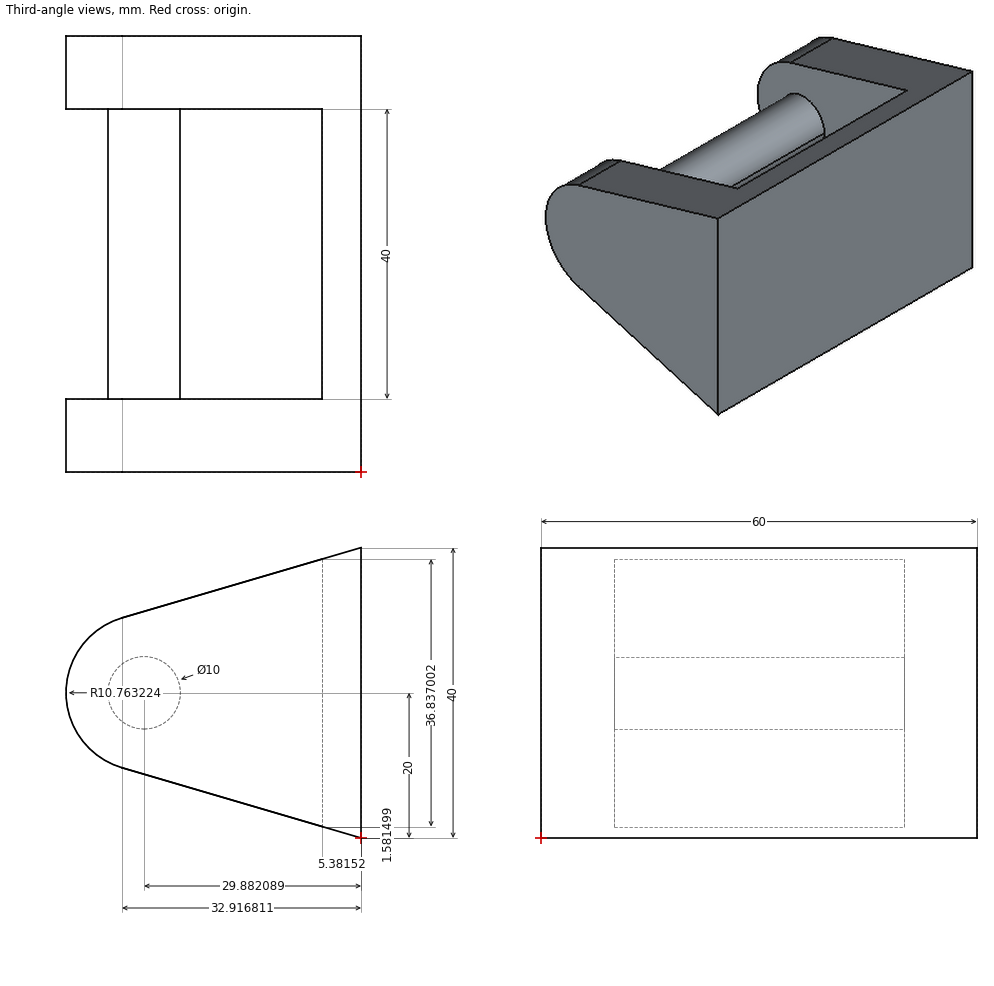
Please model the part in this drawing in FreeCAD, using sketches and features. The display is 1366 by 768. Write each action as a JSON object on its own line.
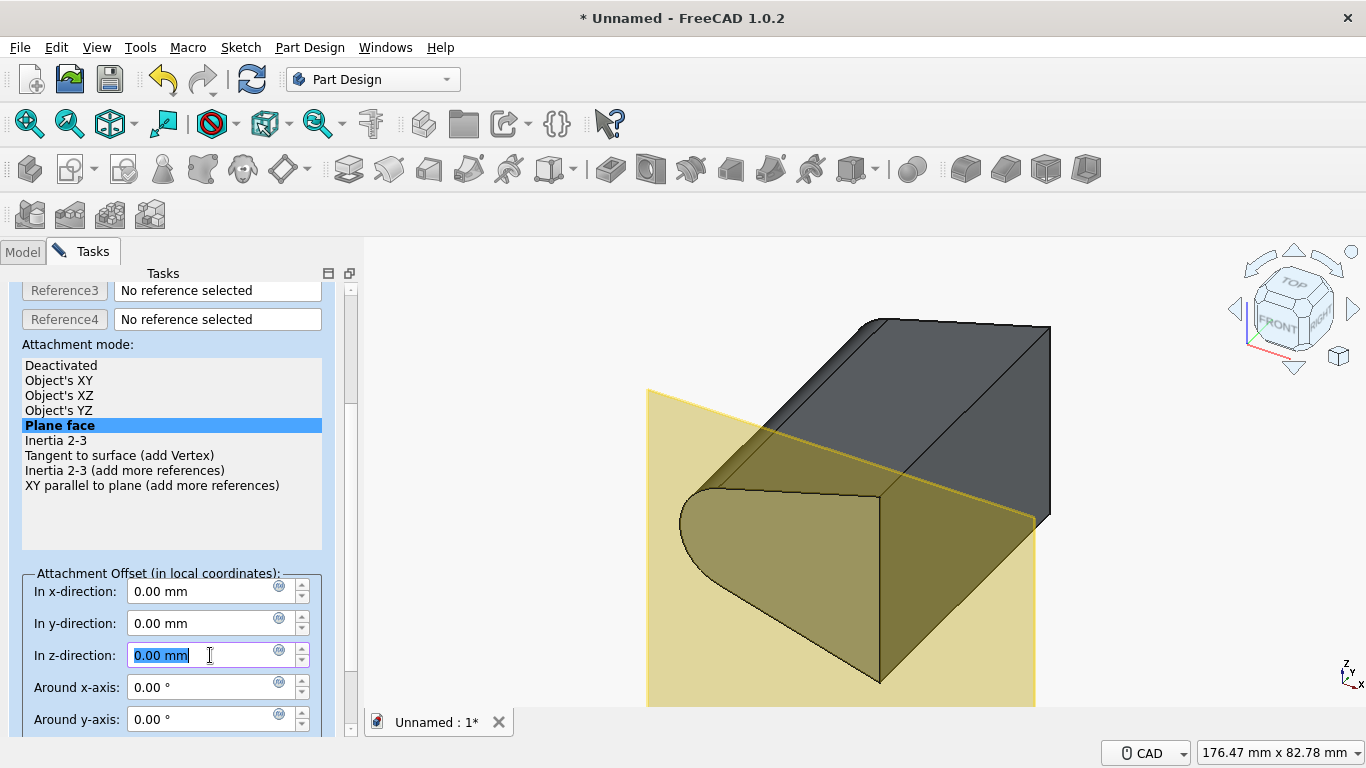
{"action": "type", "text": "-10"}
{"action": "key", "text": "Tab"}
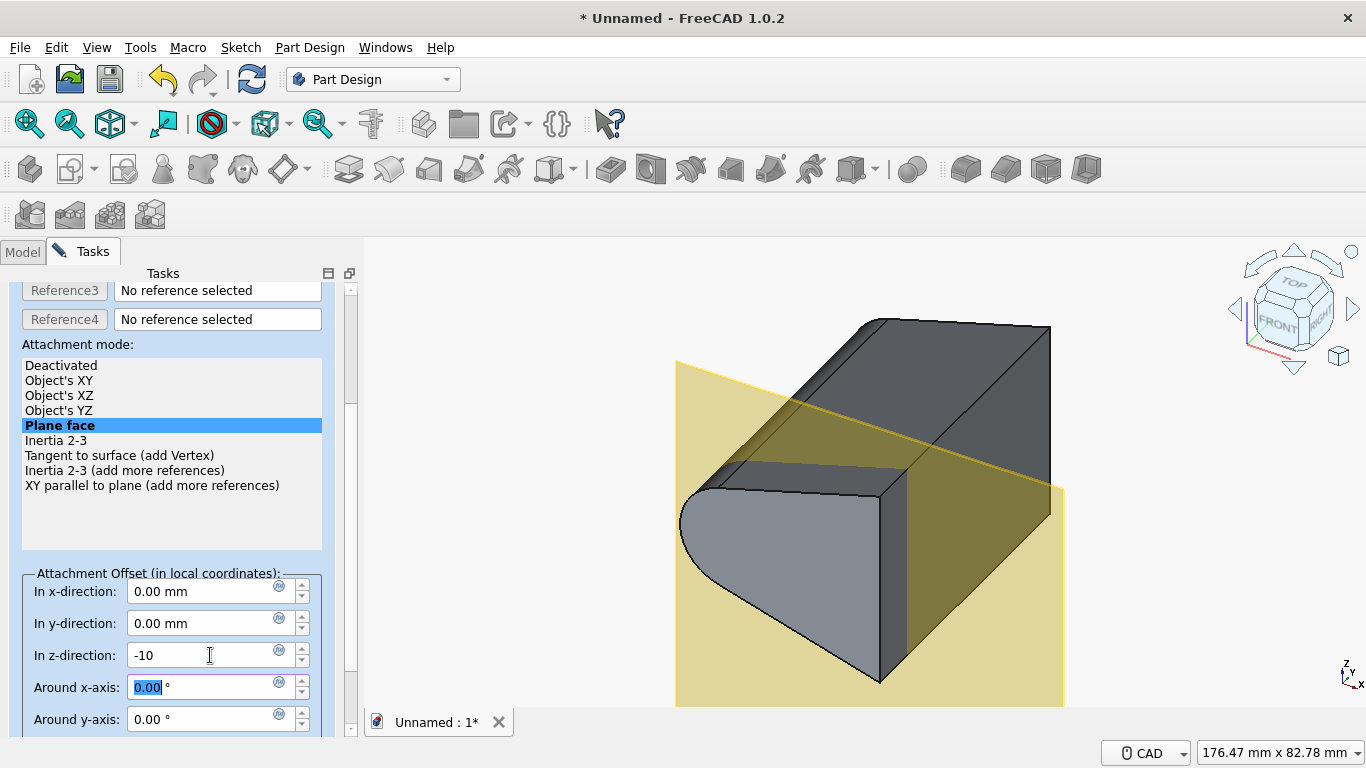
{"action": "scroll", "coordinate": [351, 510], "scroll_direction": "up", "scroll_amount": 4}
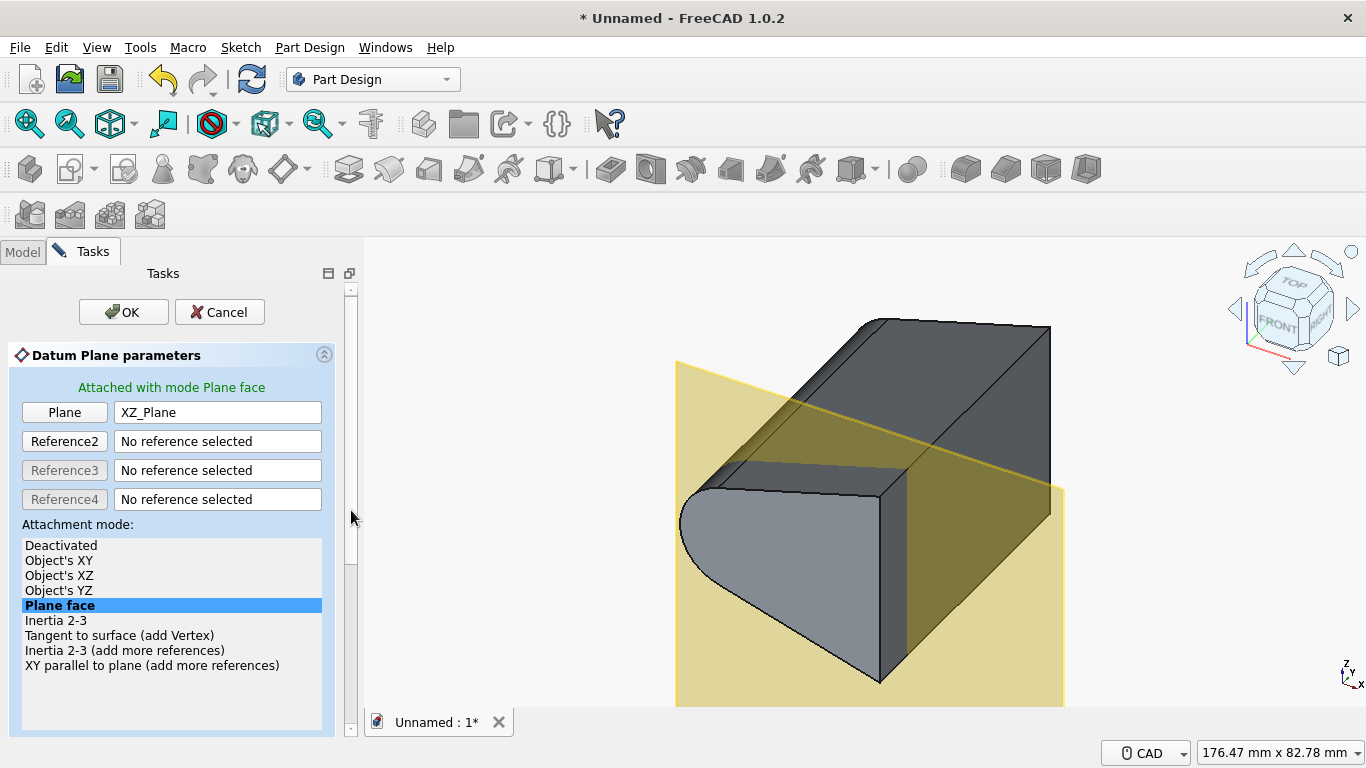
{"action": "left_click", "coordinate": [124, 312]}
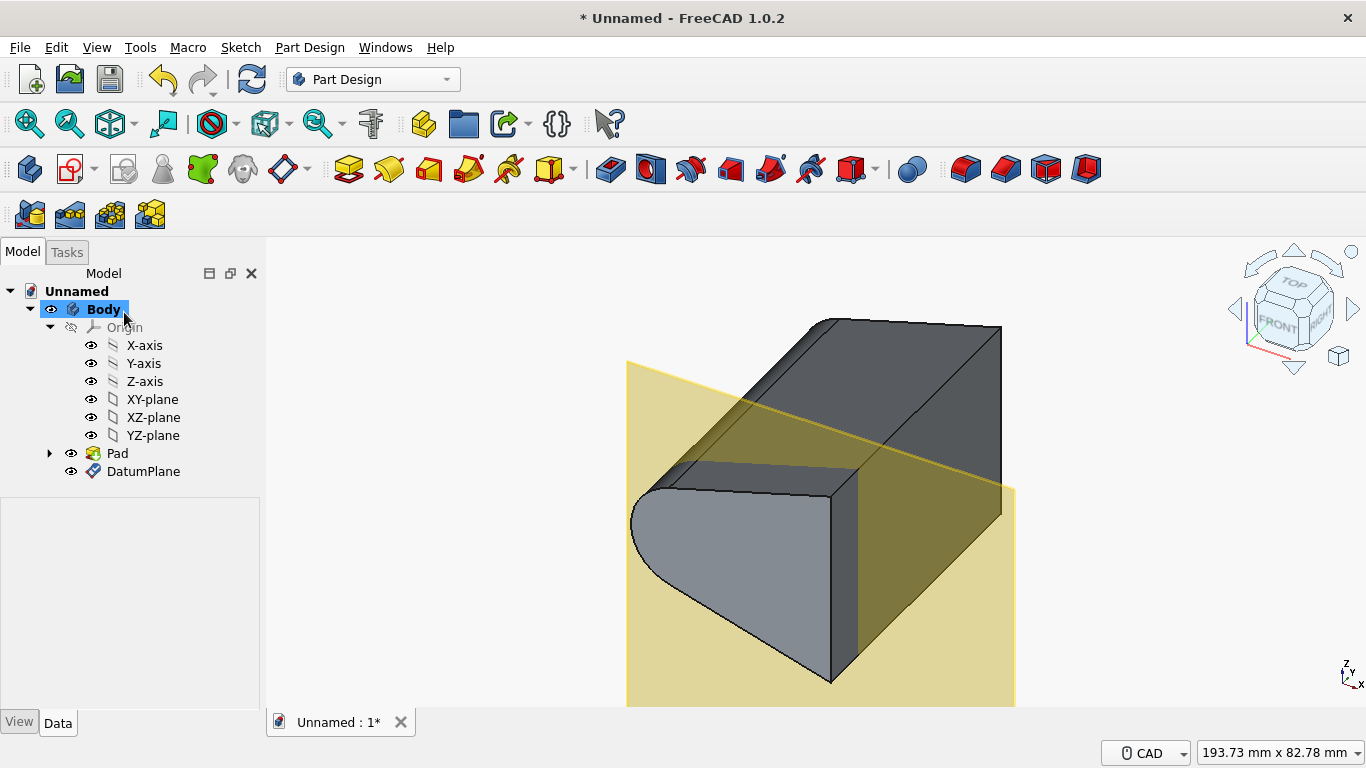
{"action": "left_click", "coordinate": [116, 471]}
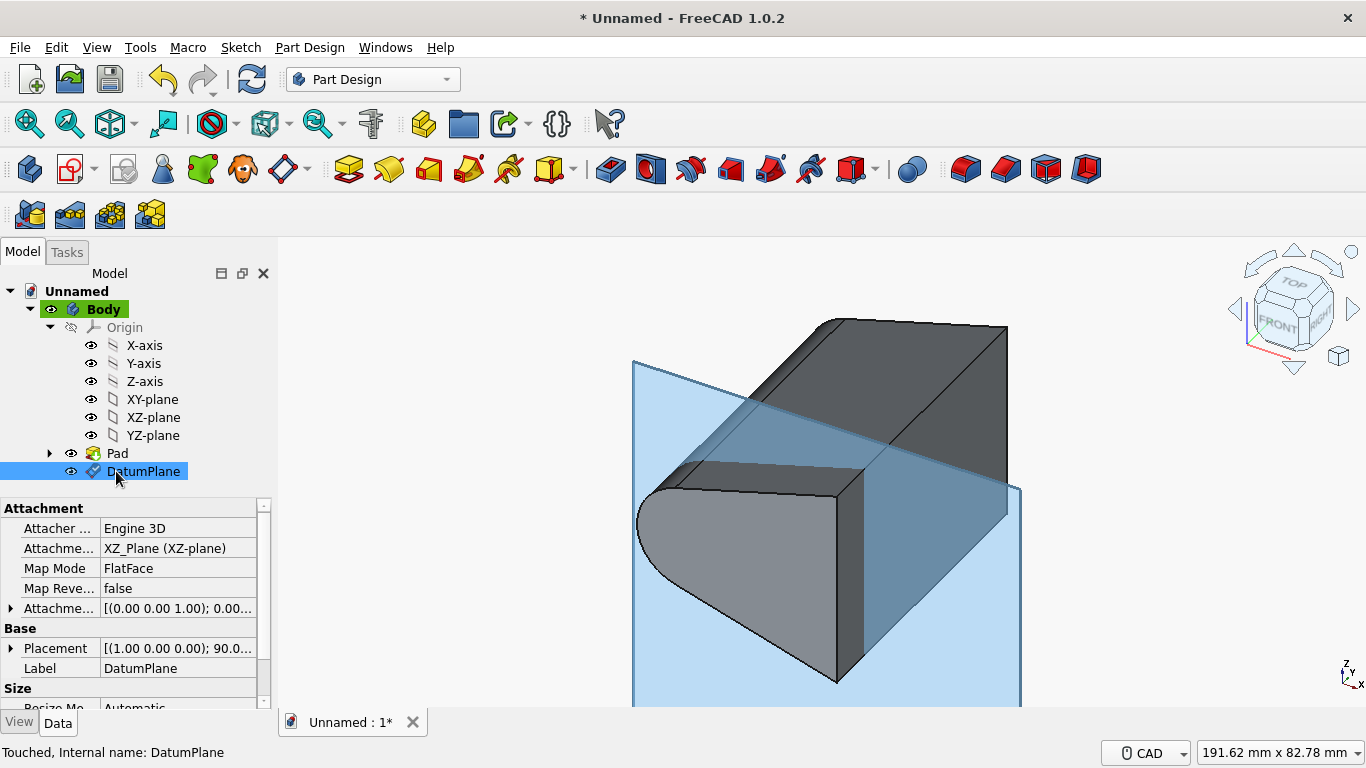
{"action": "left_click", "coordinate": [70, 170]}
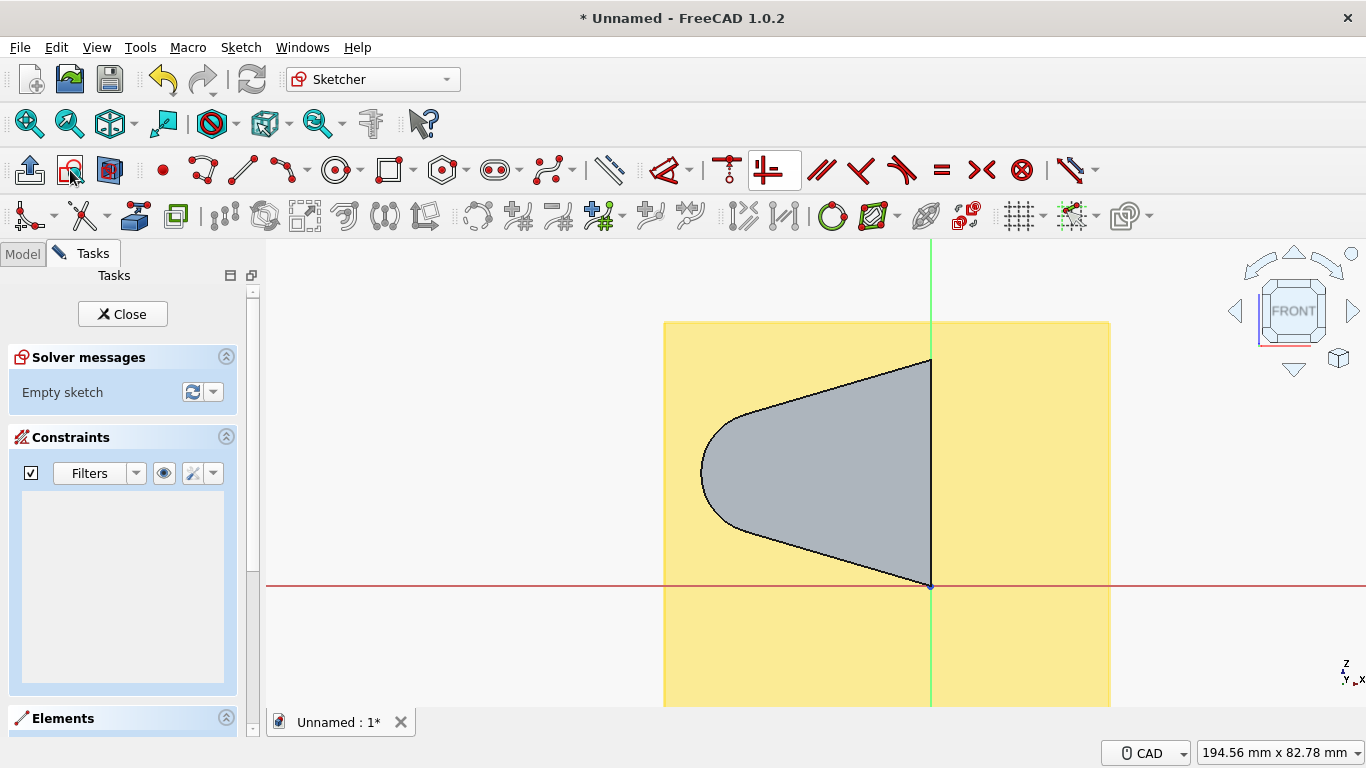
{"action": "left_click", "coordinate": [110, 170]}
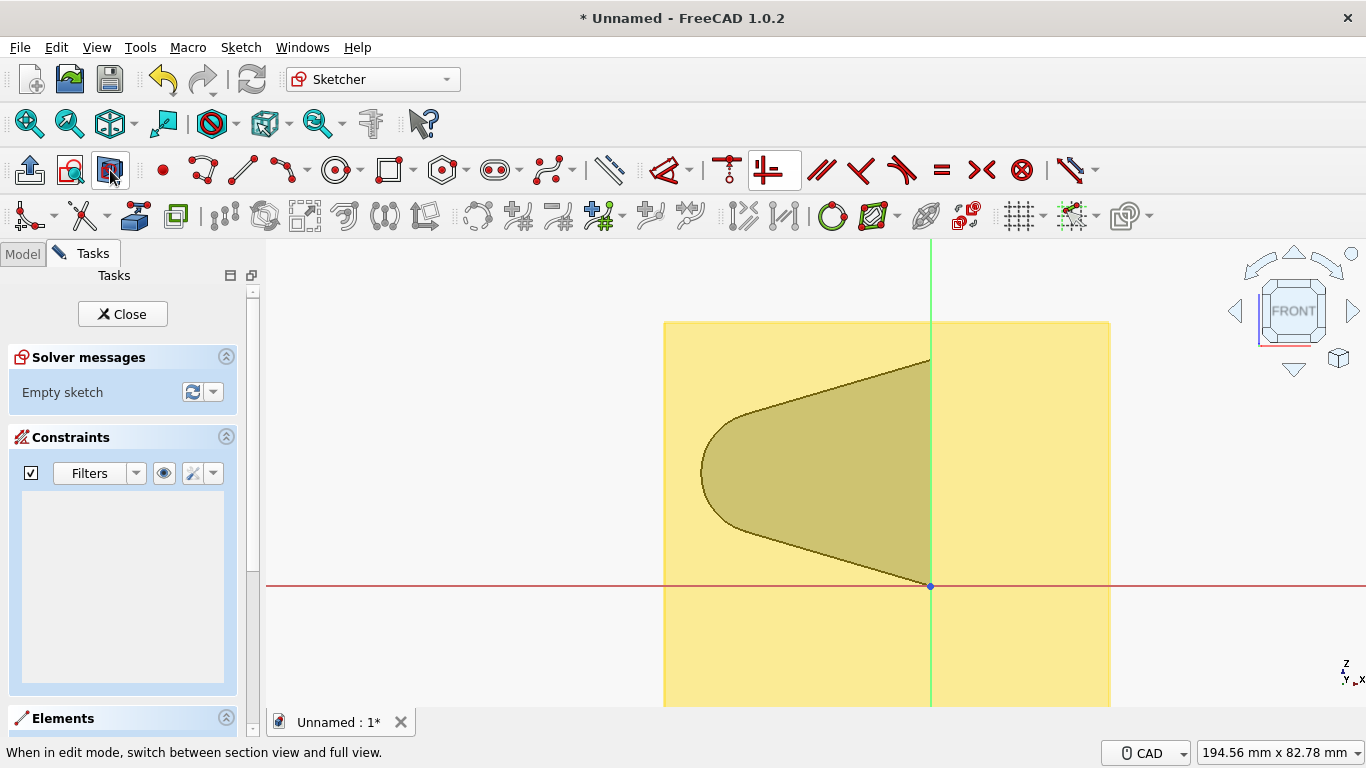
{"action": "left_click", "coordinate": [204, 170]}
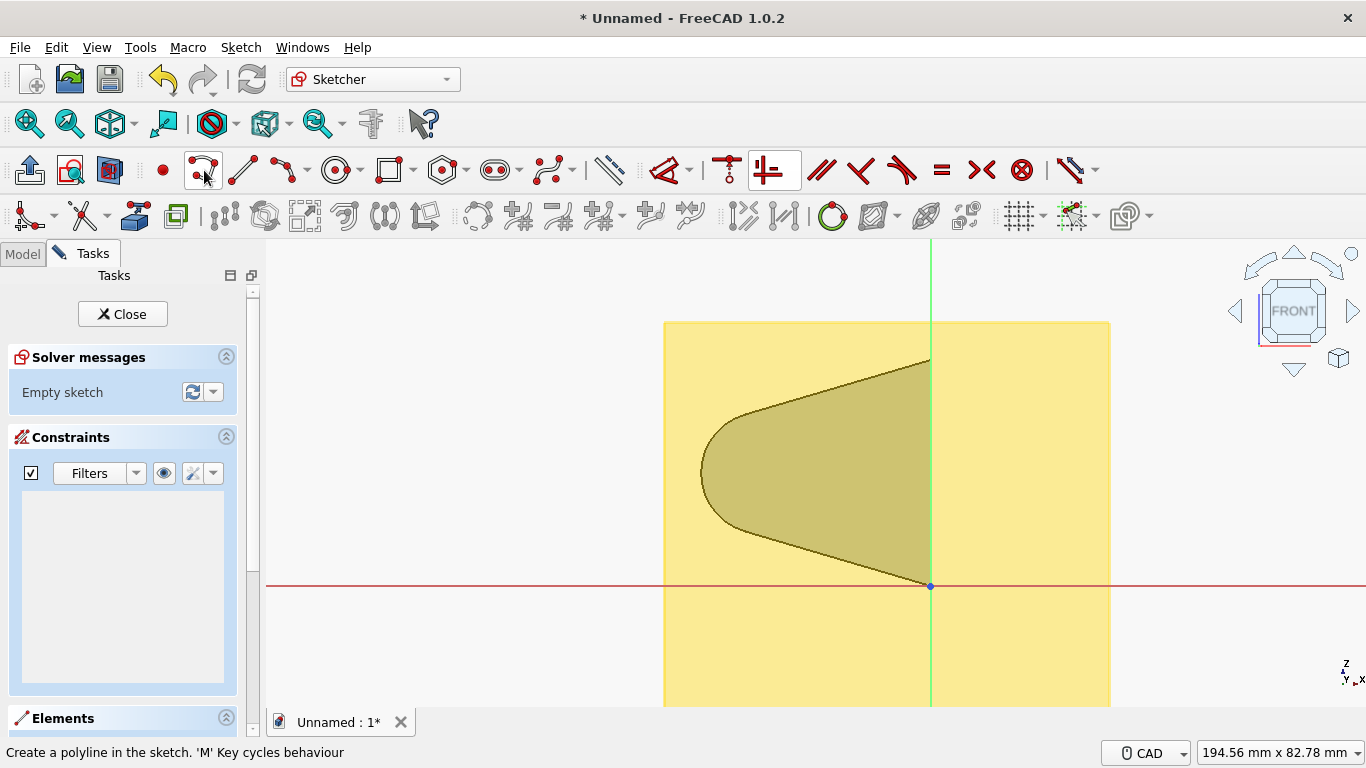
{"action": "left_click", "coordinate": [745, 531]}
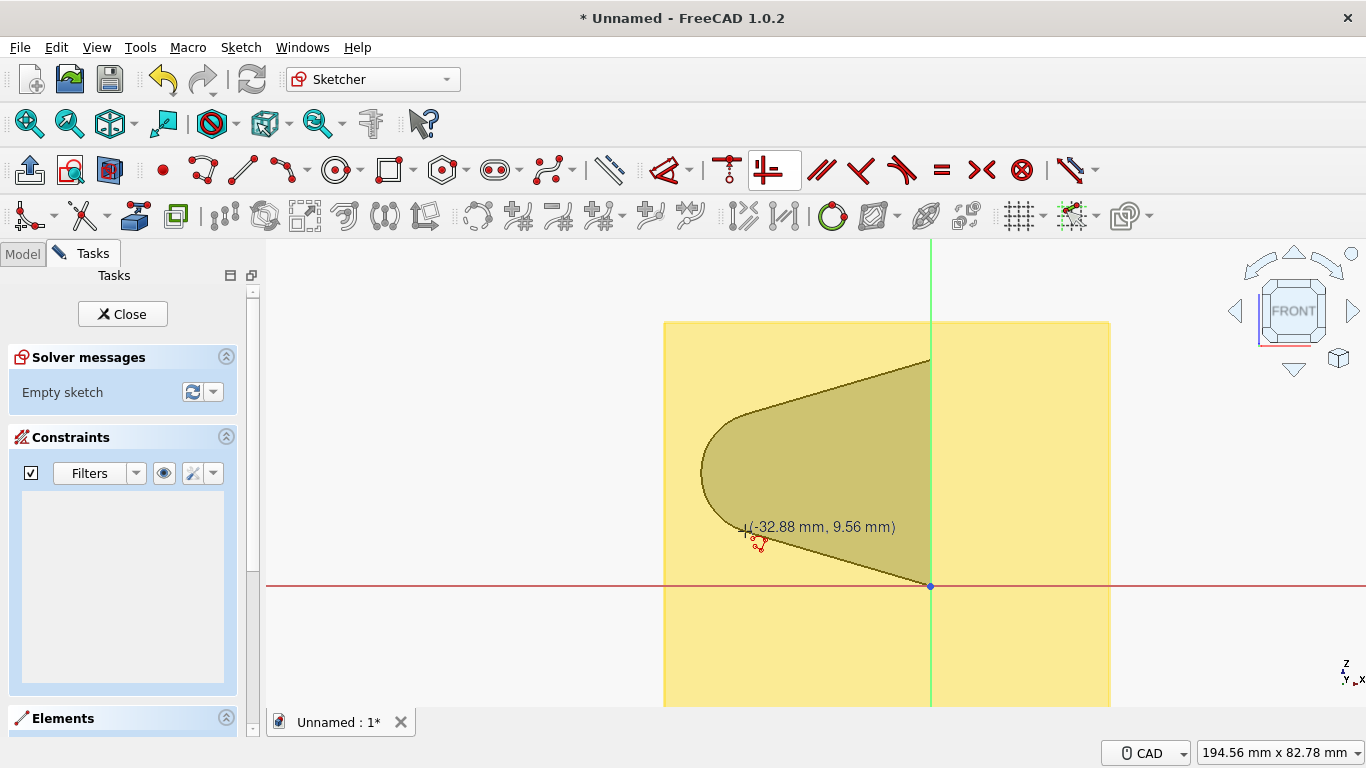
{"action": "scroll", "coordinate": [900, 577], "scroll_direction": "up", "scroll_amount": 3}